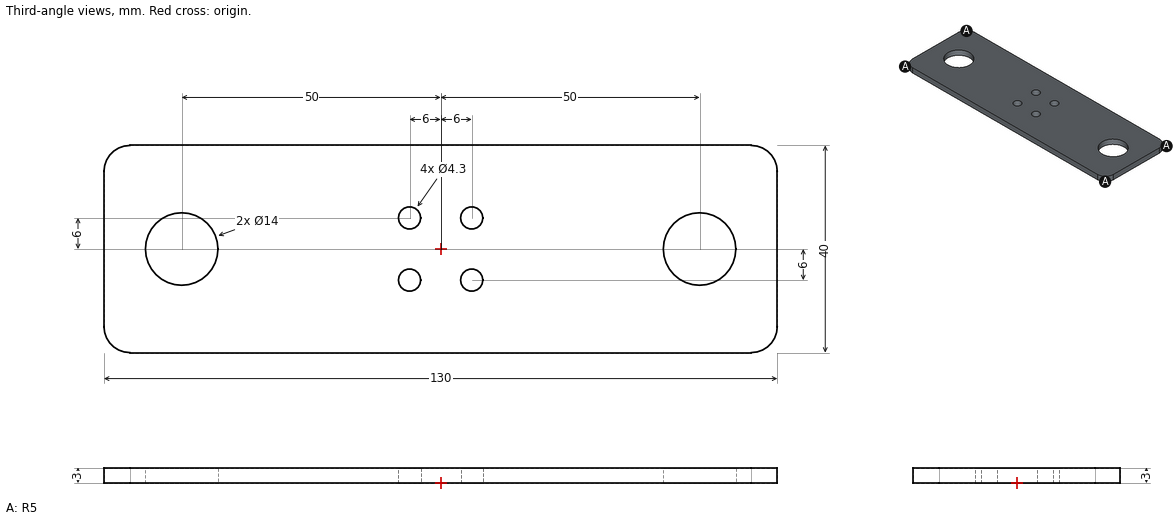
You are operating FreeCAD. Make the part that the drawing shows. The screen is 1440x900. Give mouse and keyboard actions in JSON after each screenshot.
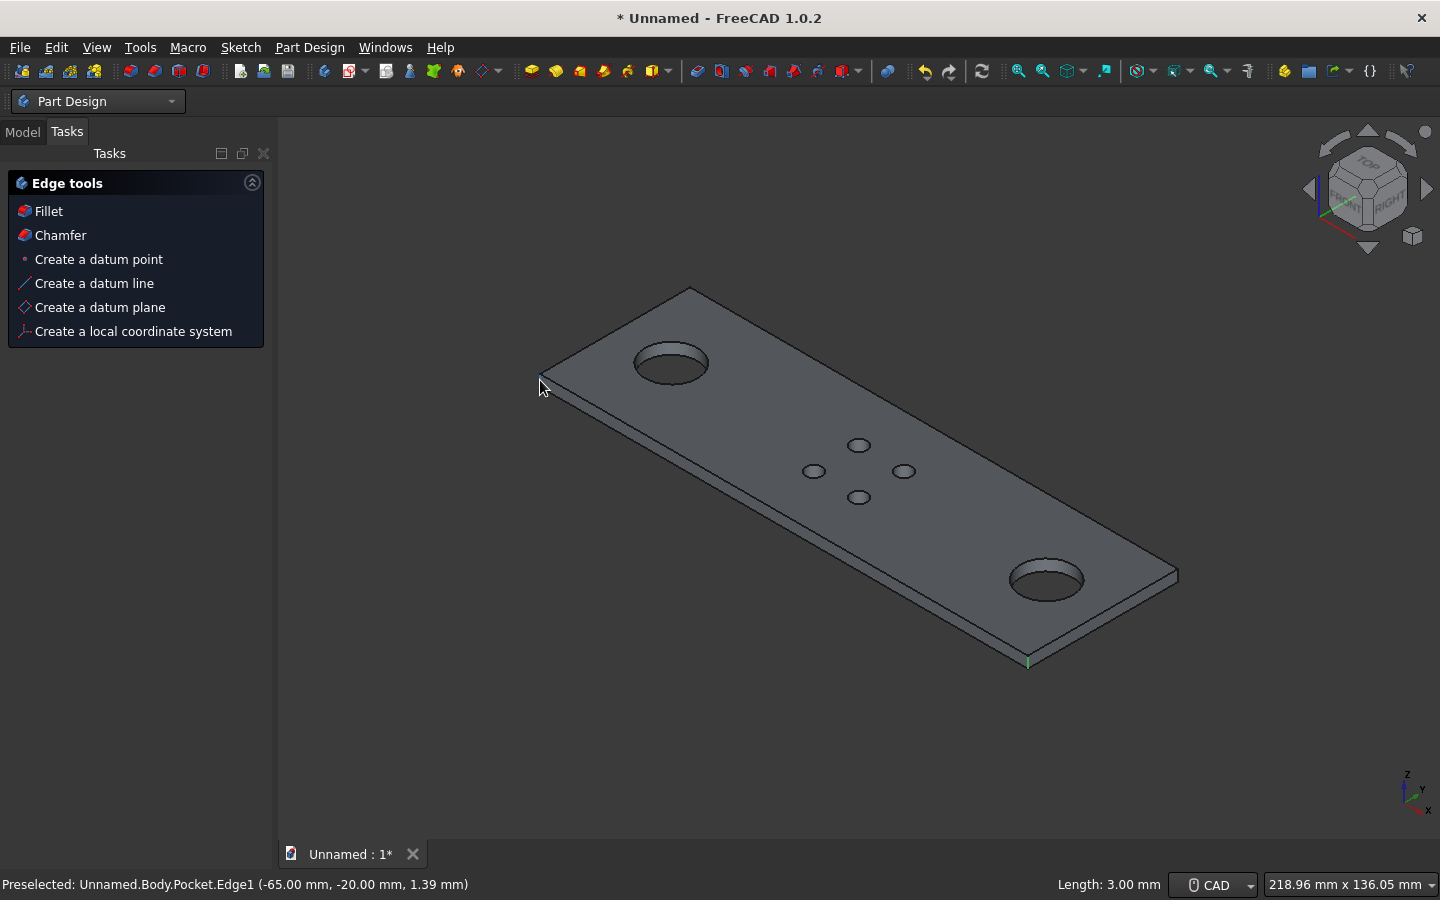
{"action": "key", "text": "2"}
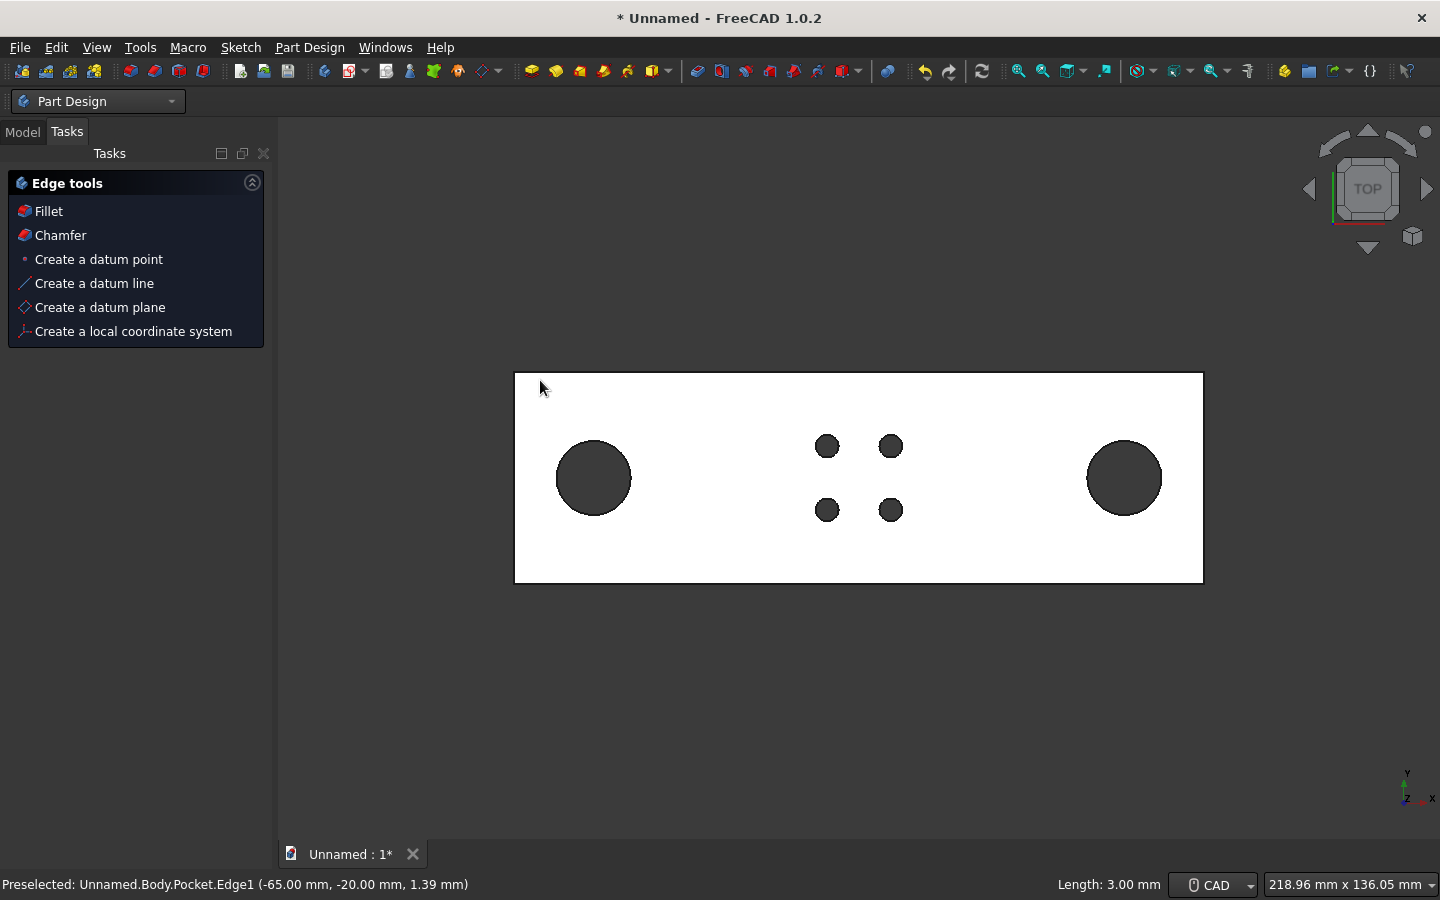
{"action": "scroll", "coordinate": [514, 583], "scroll_direction": "up", "scroll_amount": 5}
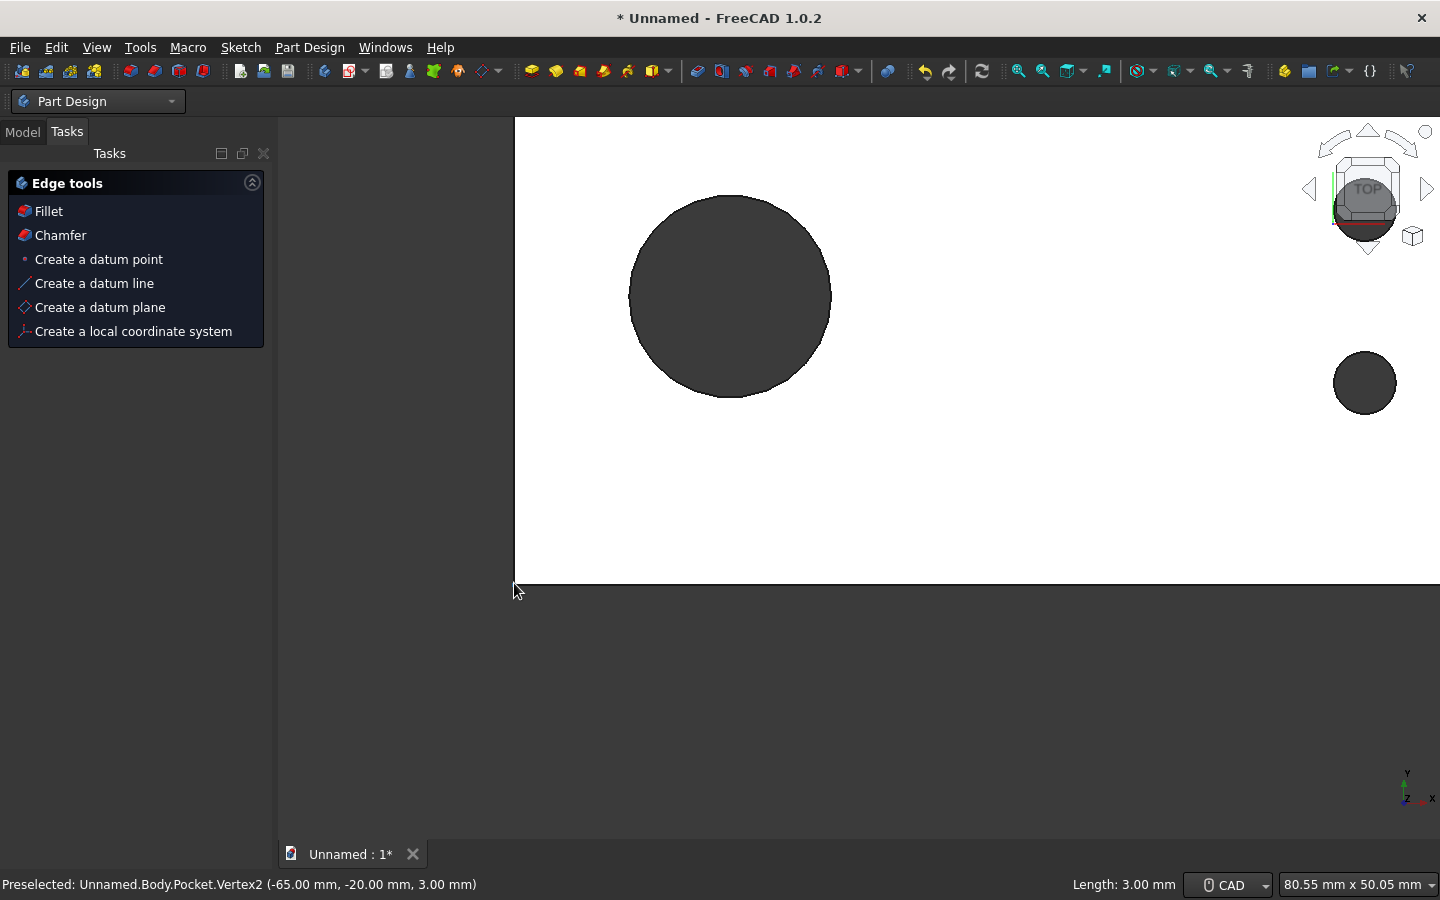
{"action": "key", "text": "v f"}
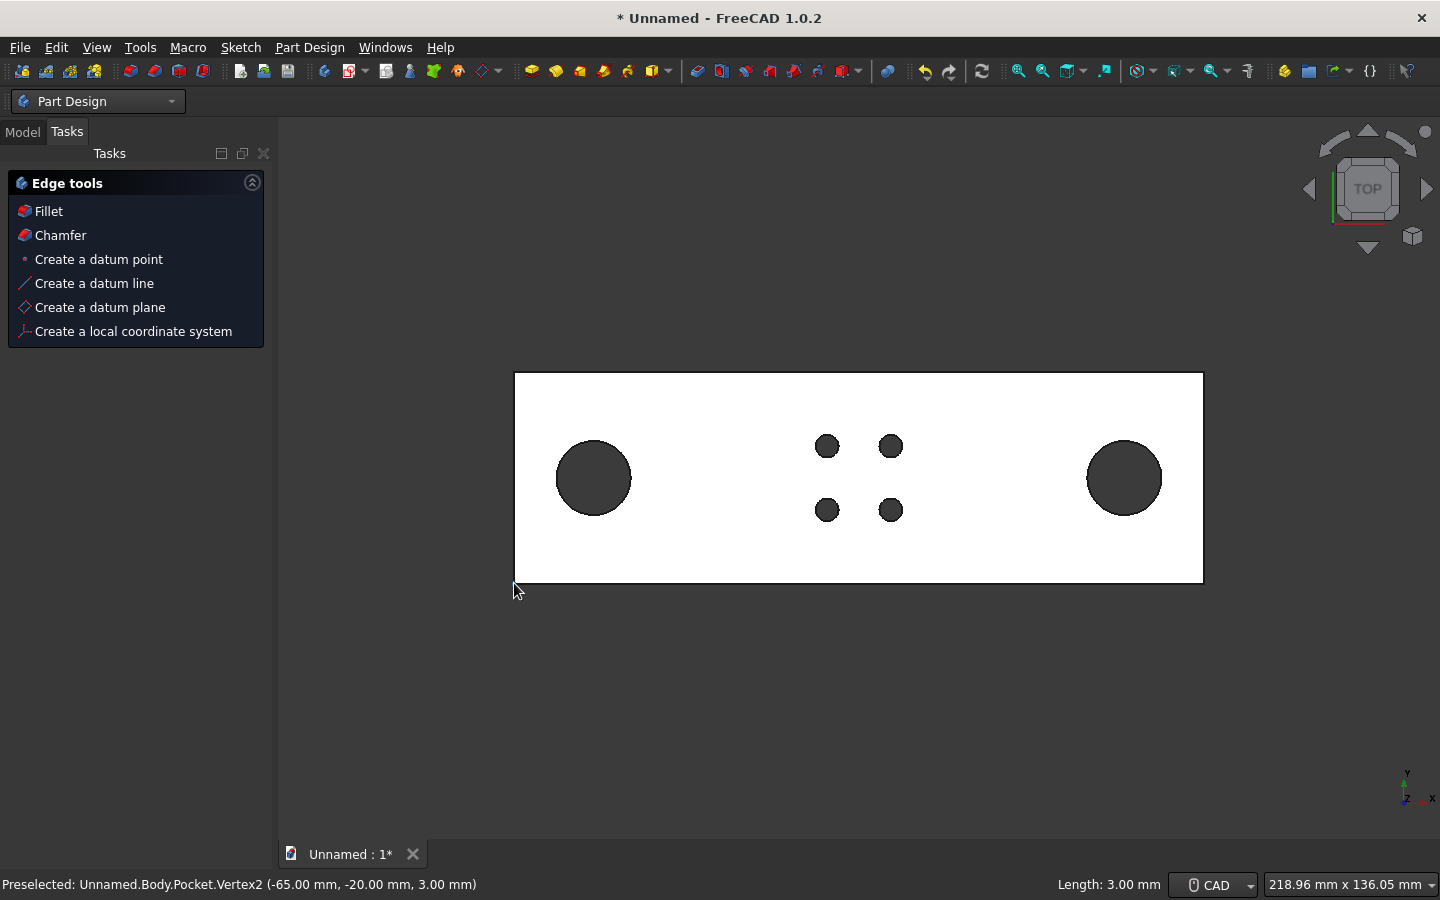
{"action": "key", "text": "1"}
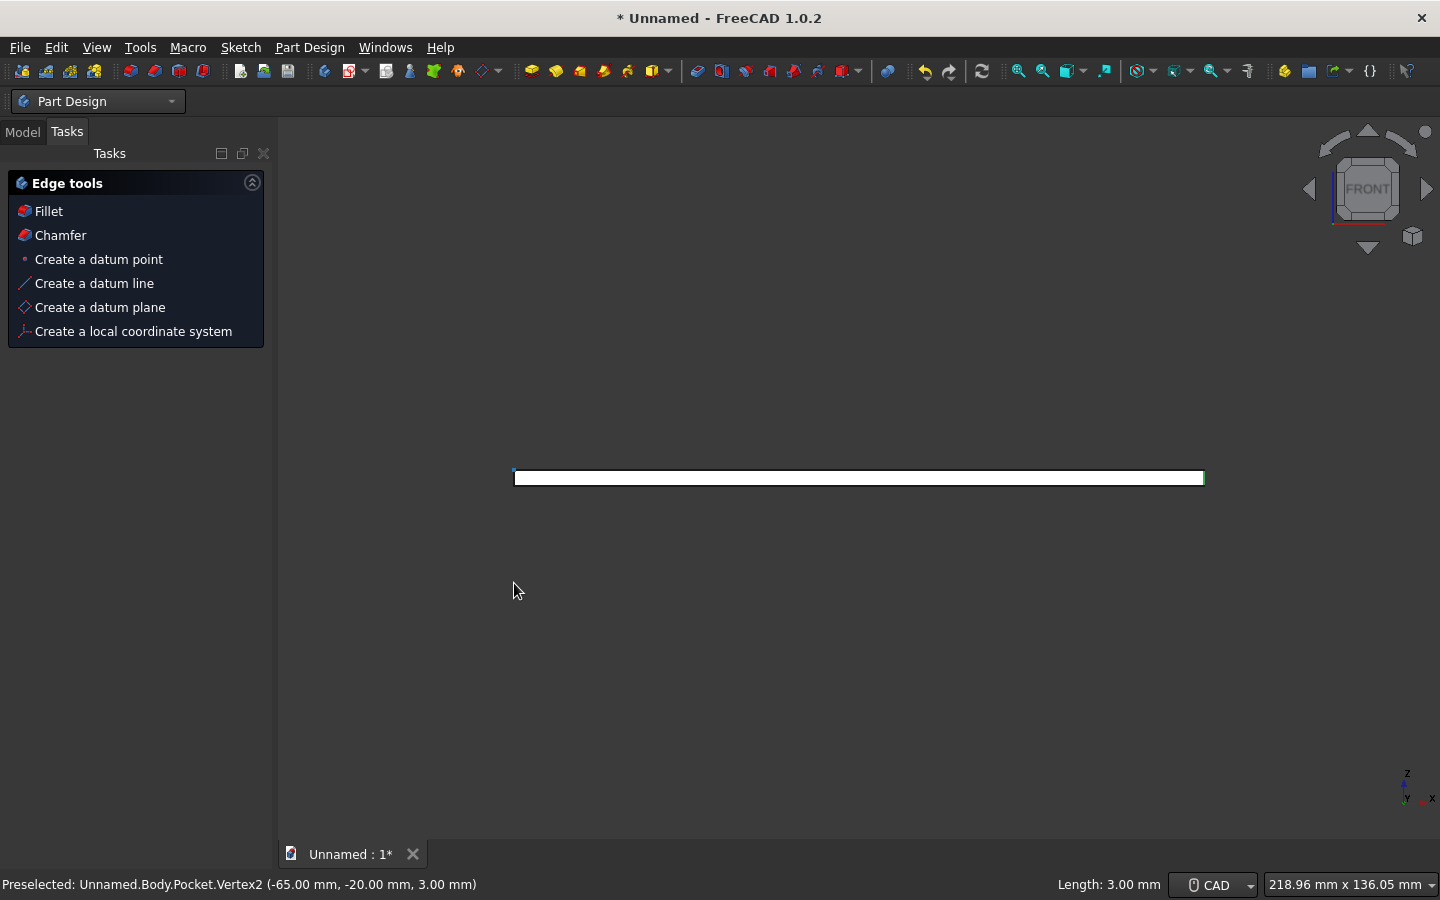
{"action": "left_click", "coordinate": [514, 477], "text": "ctrl"}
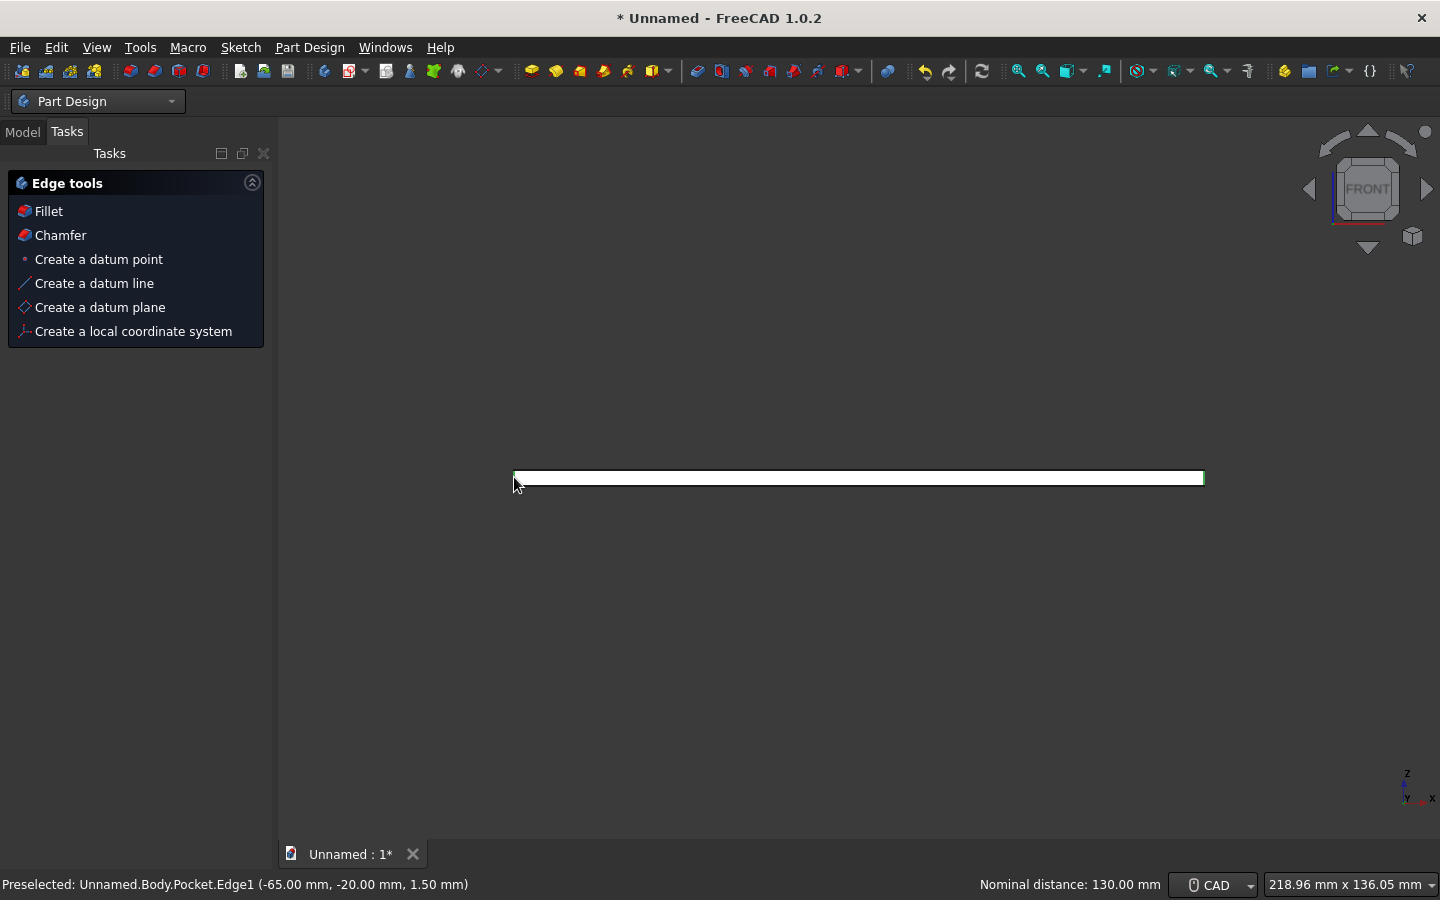
{"action": "scroll", "coordinate": [514, 477], "scroll_direction": "up", "scroll_amount": 5}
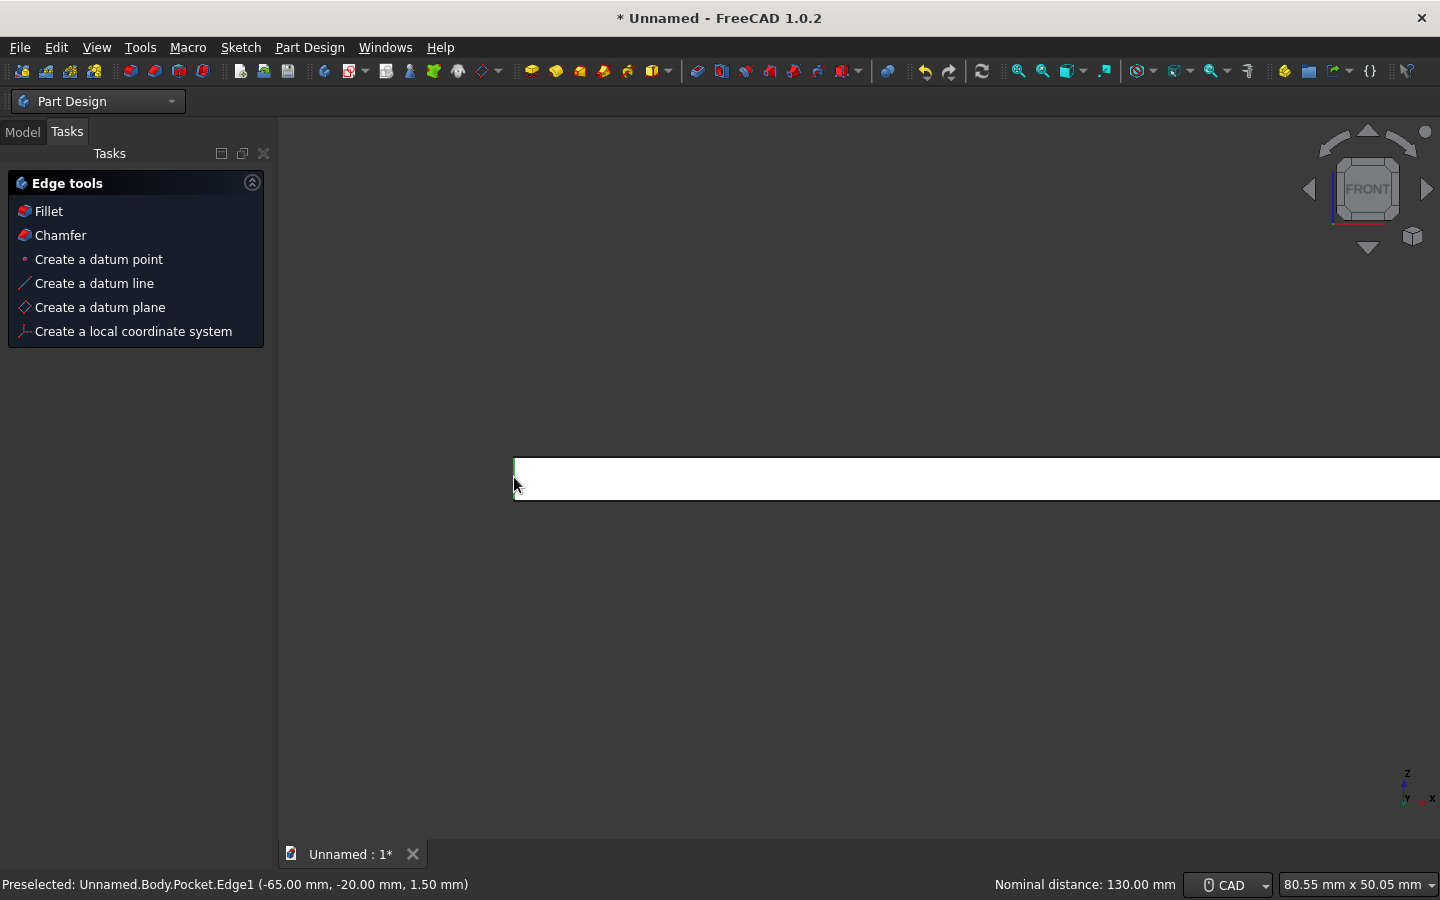
{"action": "key", "text": "v f"}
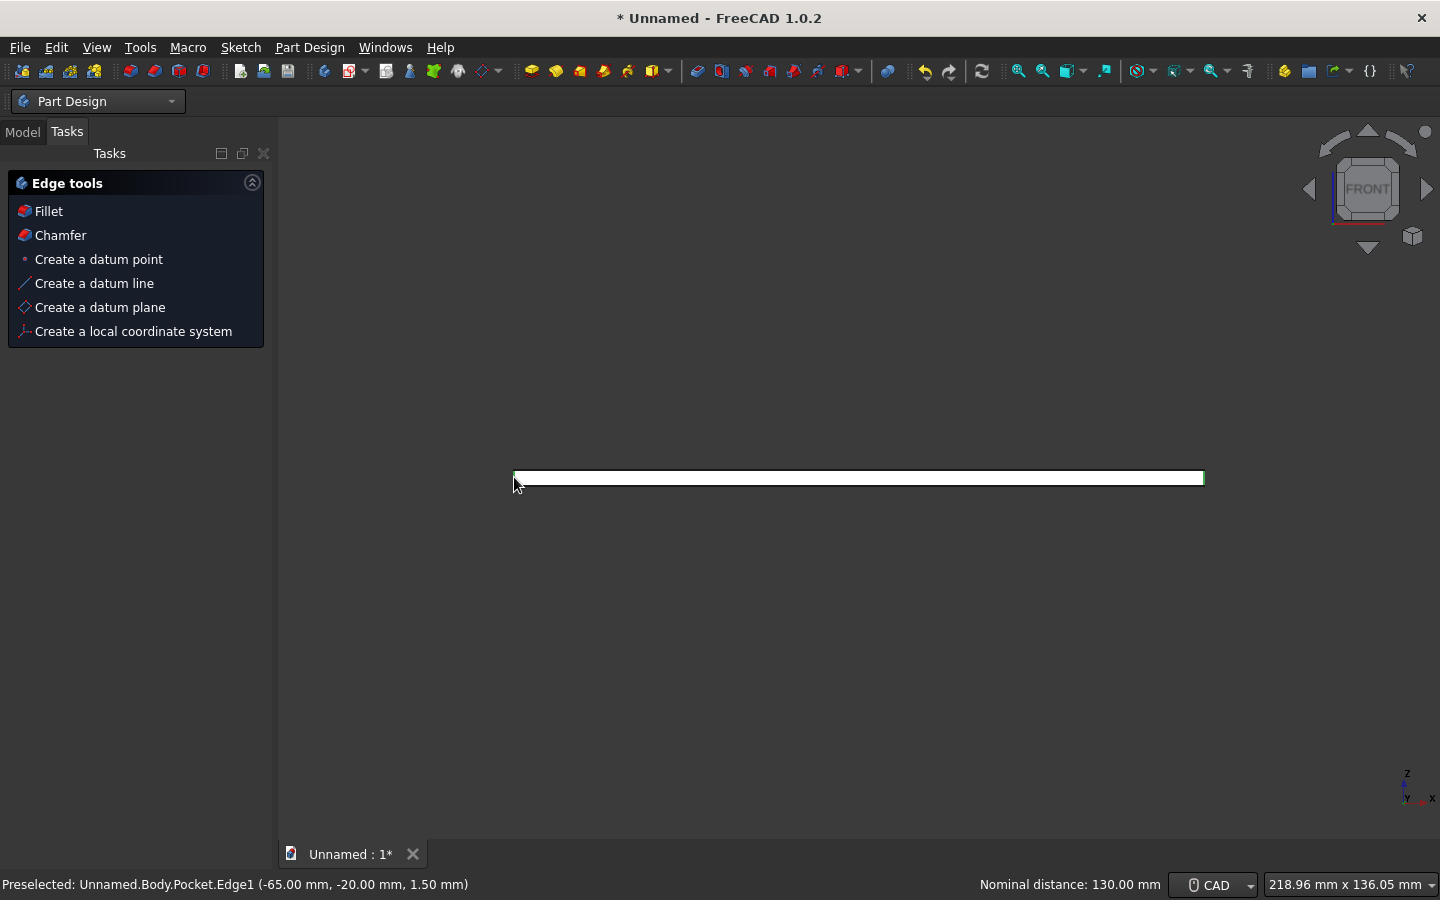
{"action": "key", "text": "3"}